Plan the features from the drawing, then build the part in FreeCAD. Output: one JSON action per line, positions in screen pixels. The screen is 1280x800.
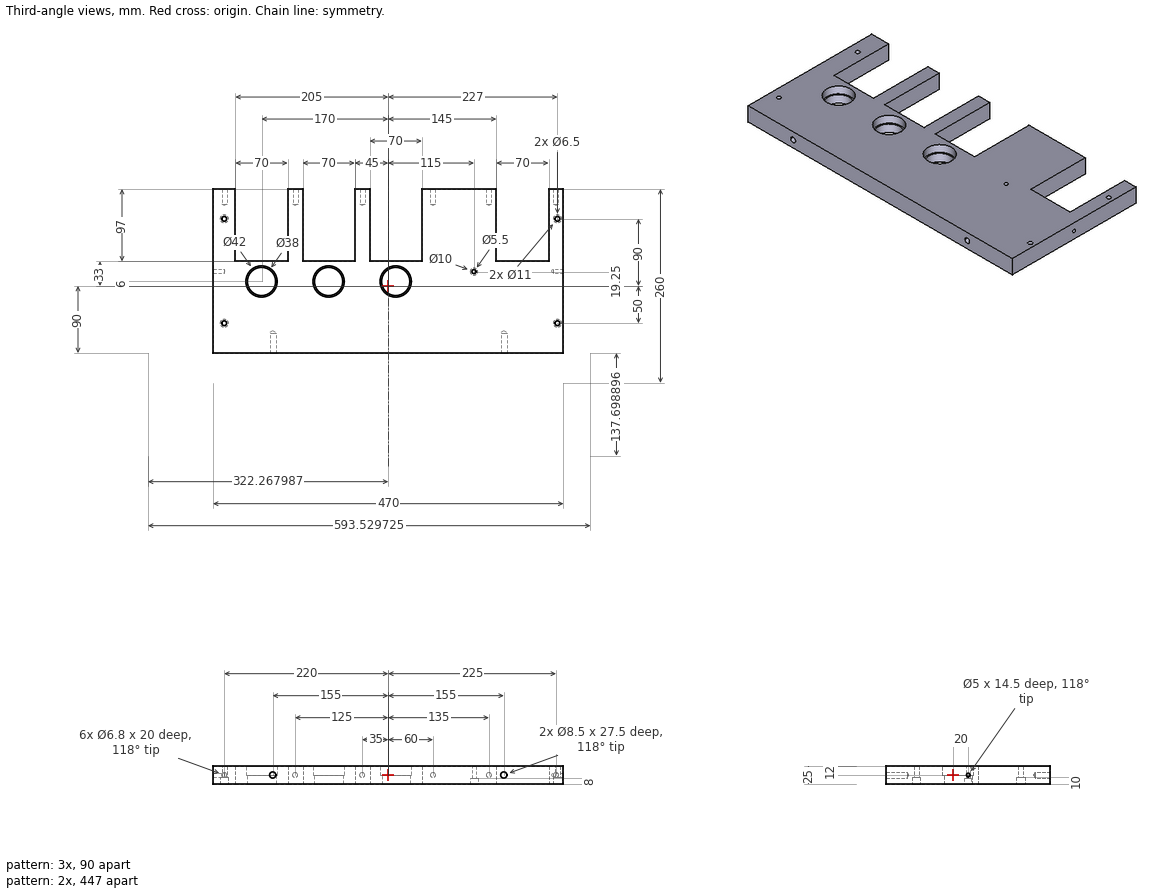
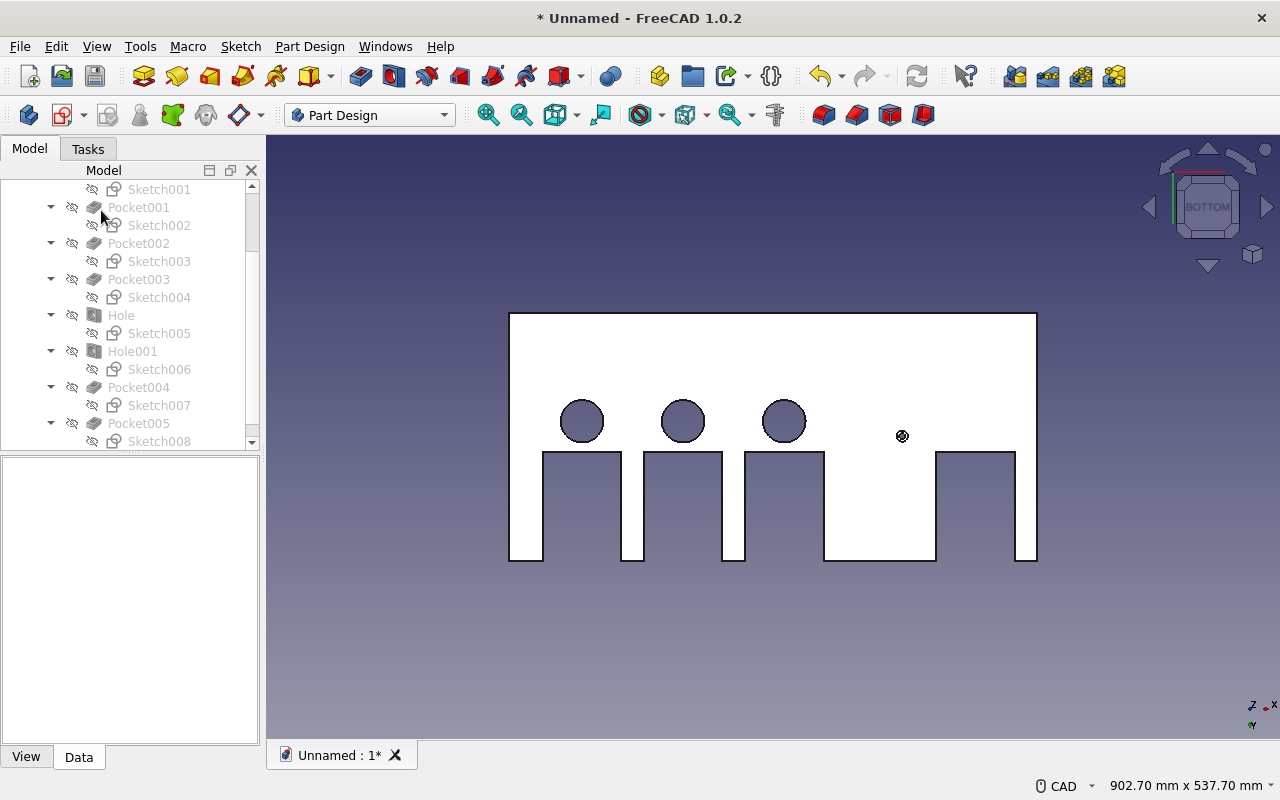
{"action": "left_click", "coordinate": [924, 365]}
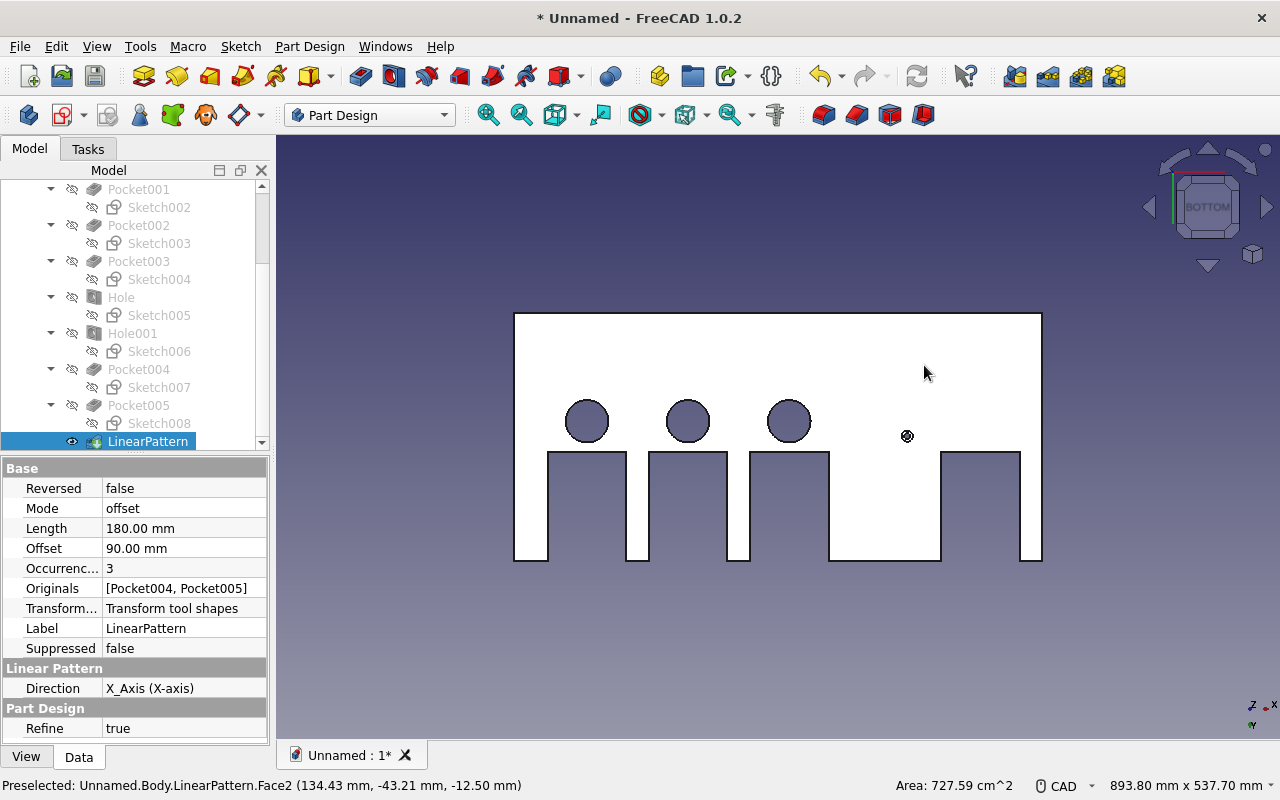
{"action": "left_click", "coordinate": [62, 116]}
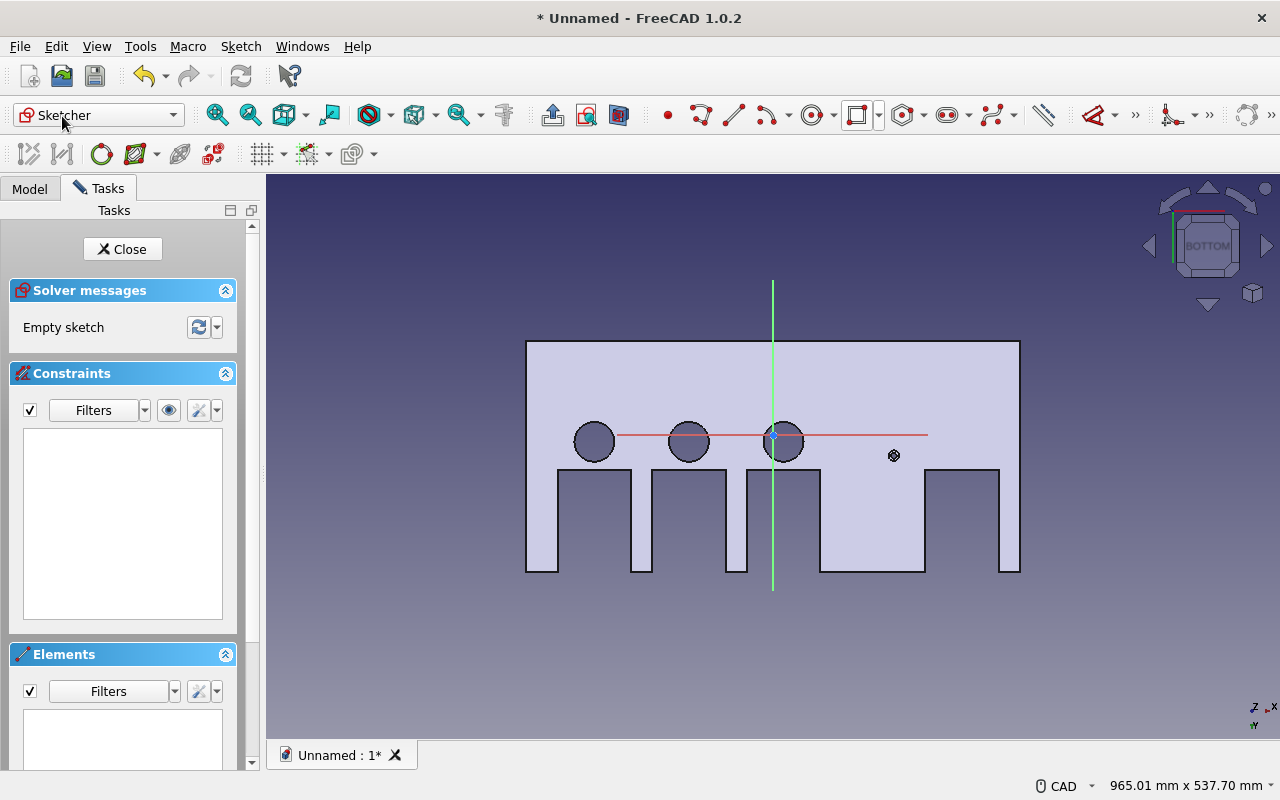
{"action": "scroll", "coordinate": [1049, 457], "scroll_direction": "up", "scroll_amount": 4}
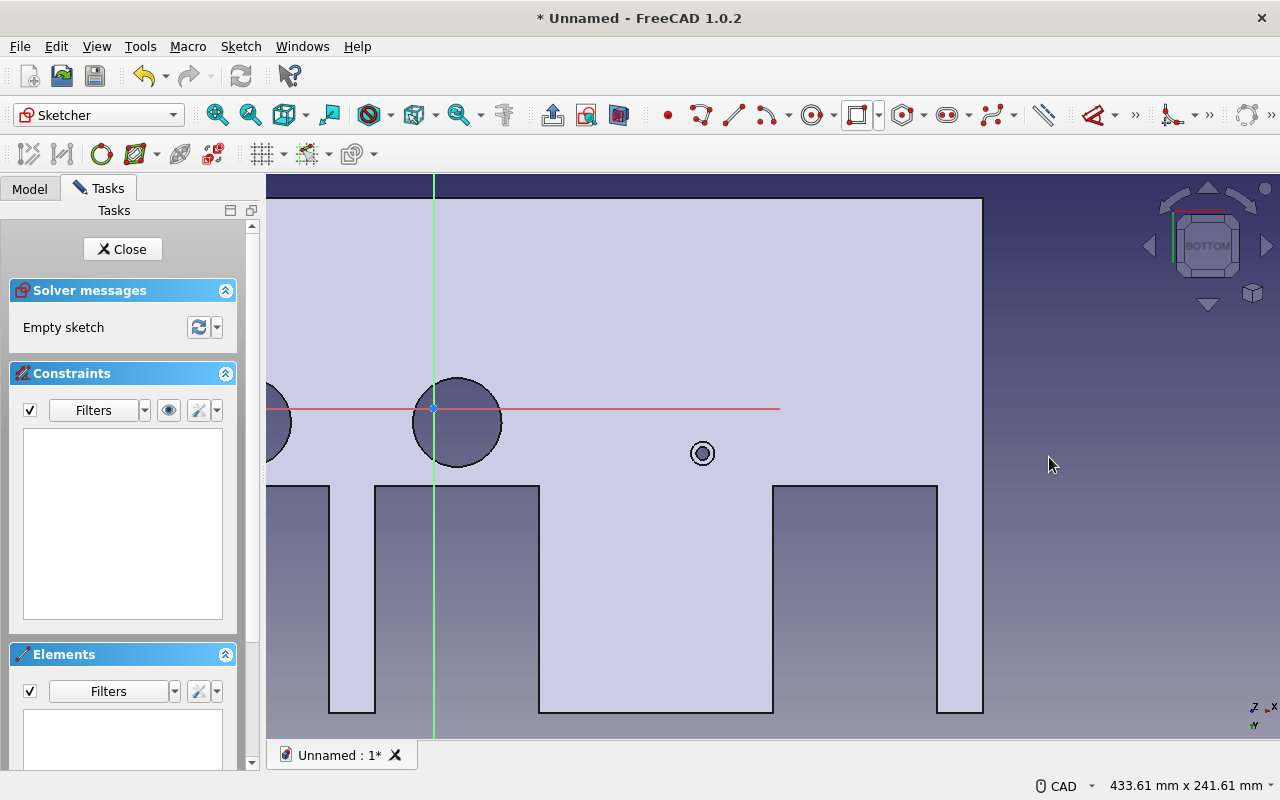
{"action": "left_click", "coordinate": [812, 116]}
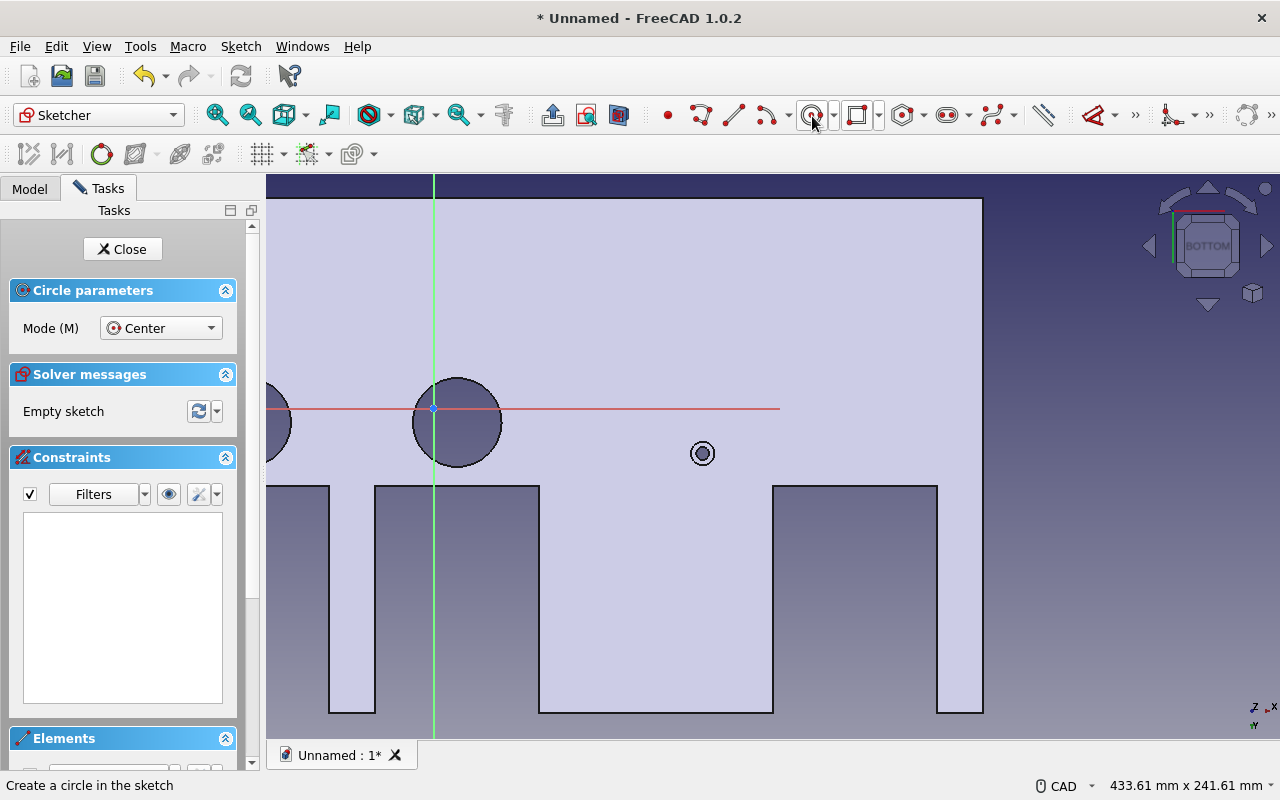
{"action": "scroll", "coordinate": [965, 619], "scroll_direction": "up", "scroll_amount": 6}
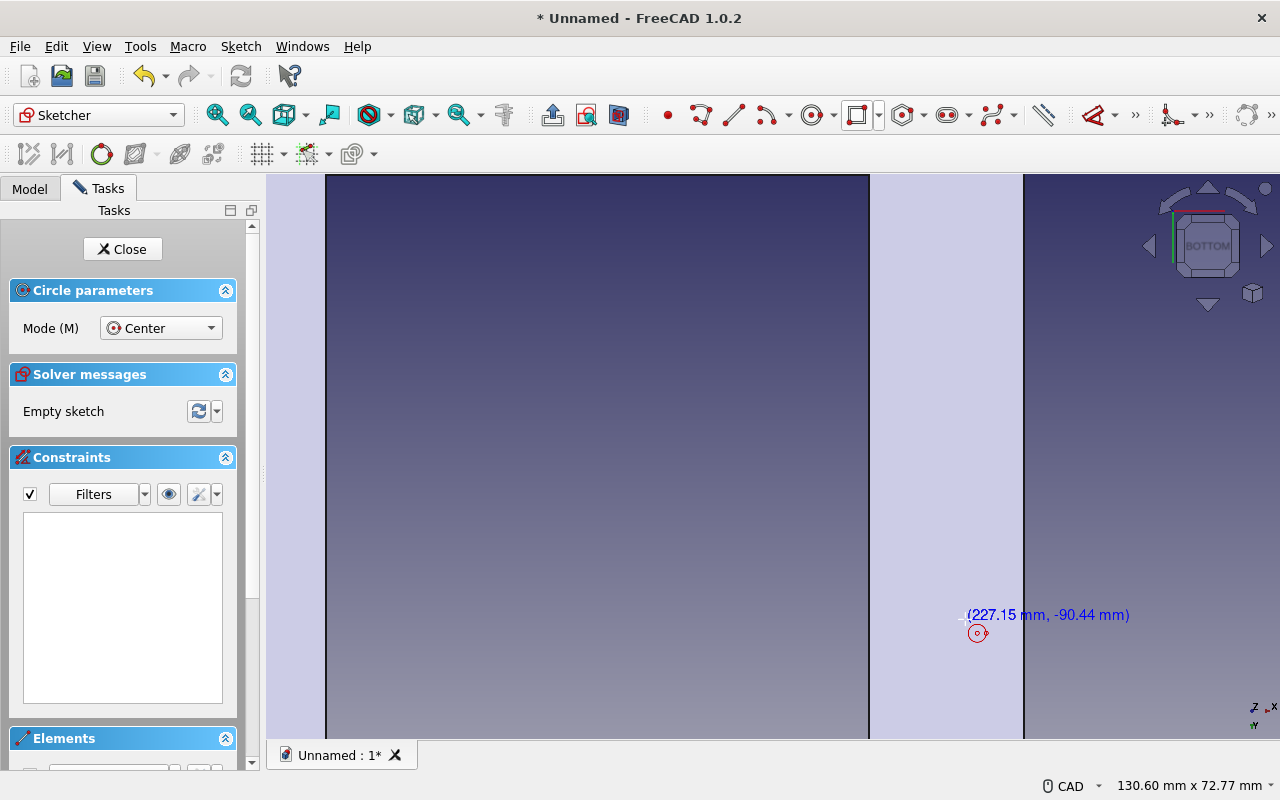
{"action": "left_click", "coordinate": [962, 617]}
{"action": "mouse_move", "coordinate": [980, 599]}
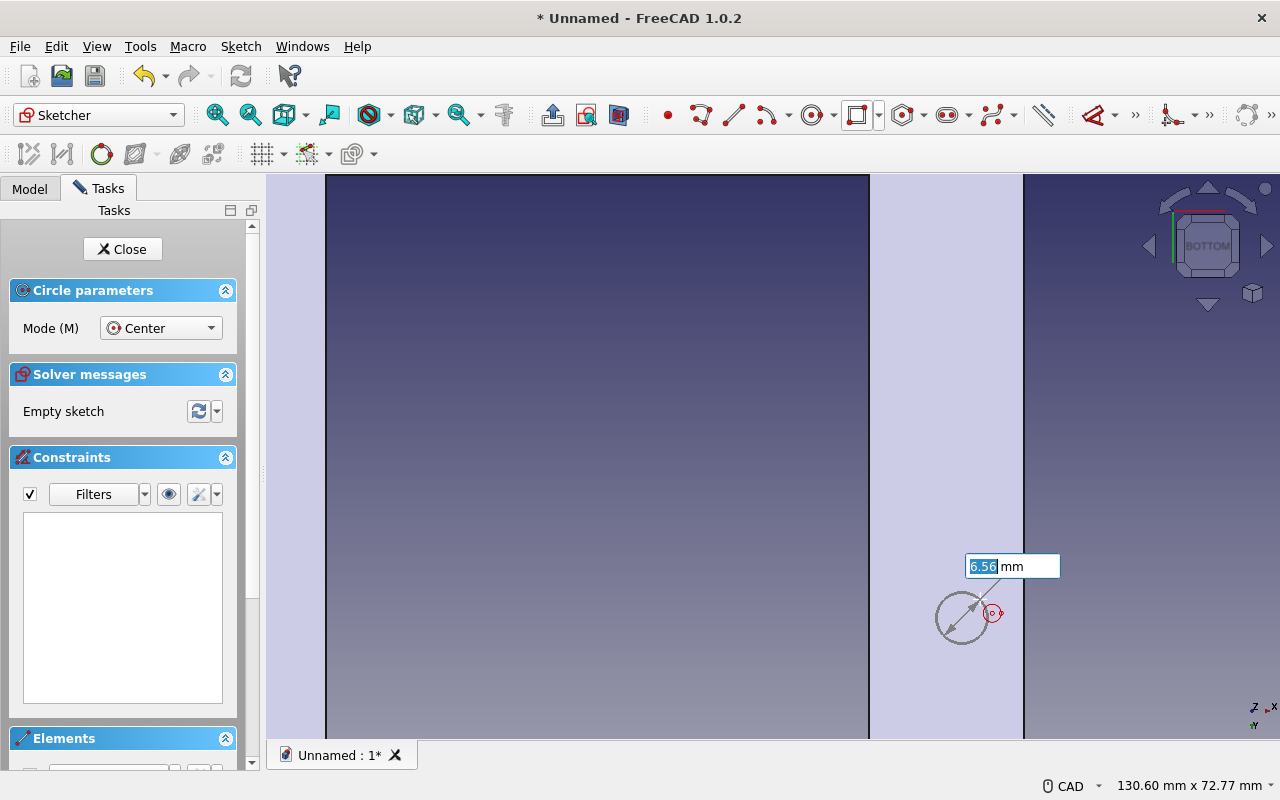
{"action": "type", "text": "6.5"}
{"action": "key", "text": "Return"}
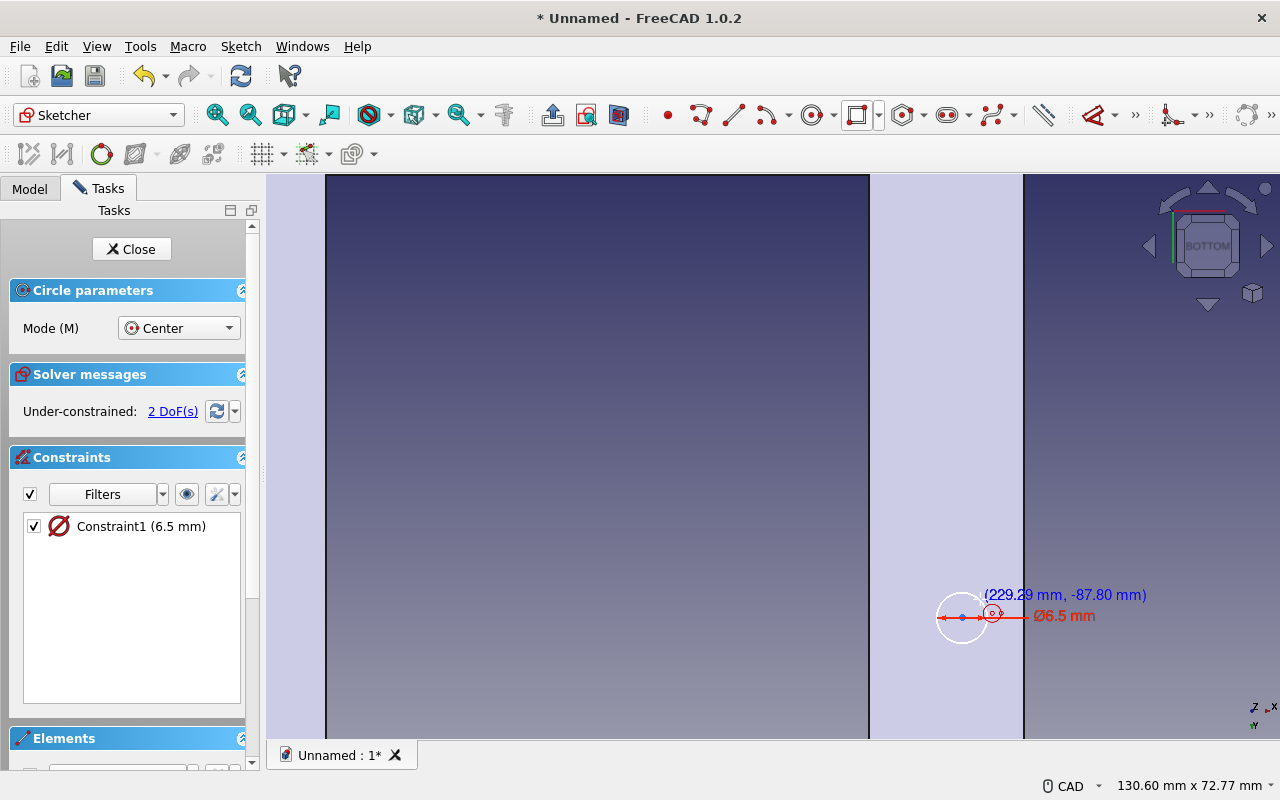
{"action": "scroll", "coordinate": [968, 622], "scroll_direction": "down", "scroll_amount": 6}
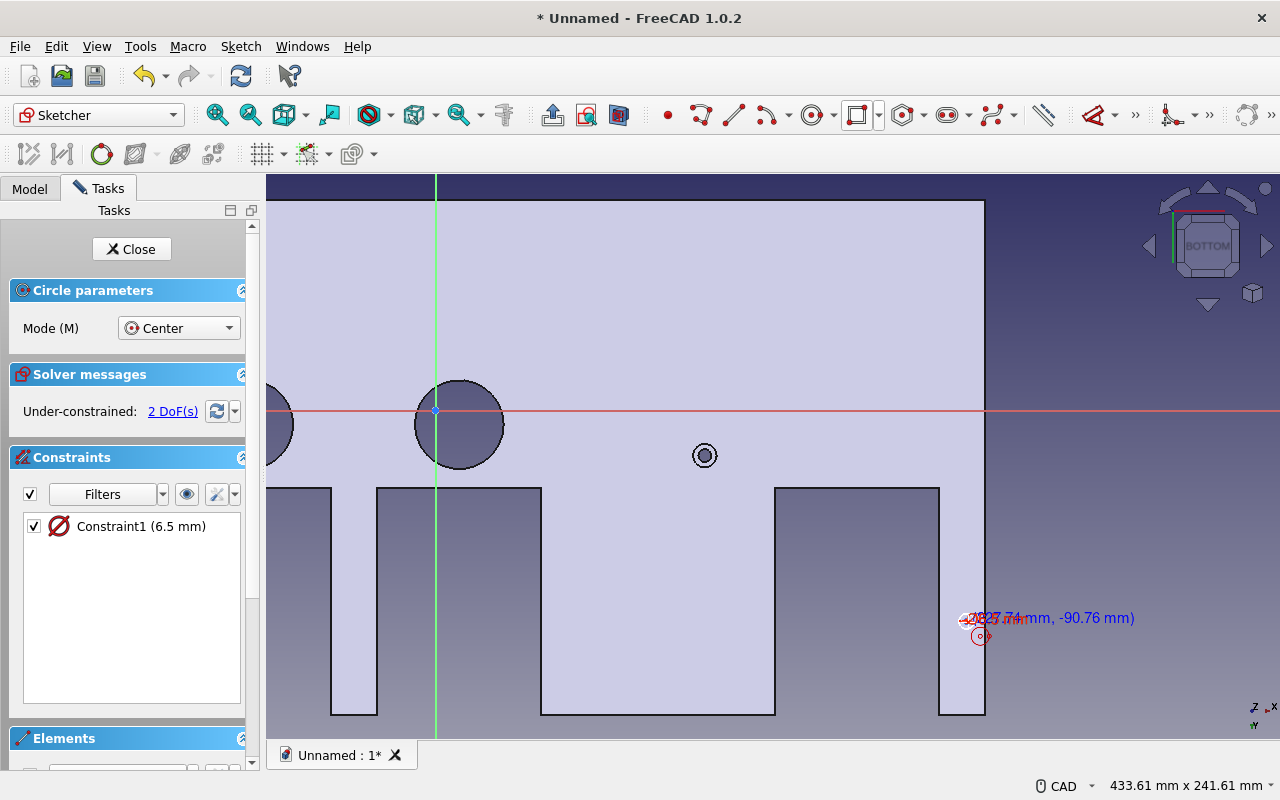
{"action": "scroll", "coordinate": [967, 294], "scroll_direction": "up", "scroll_amount": 6}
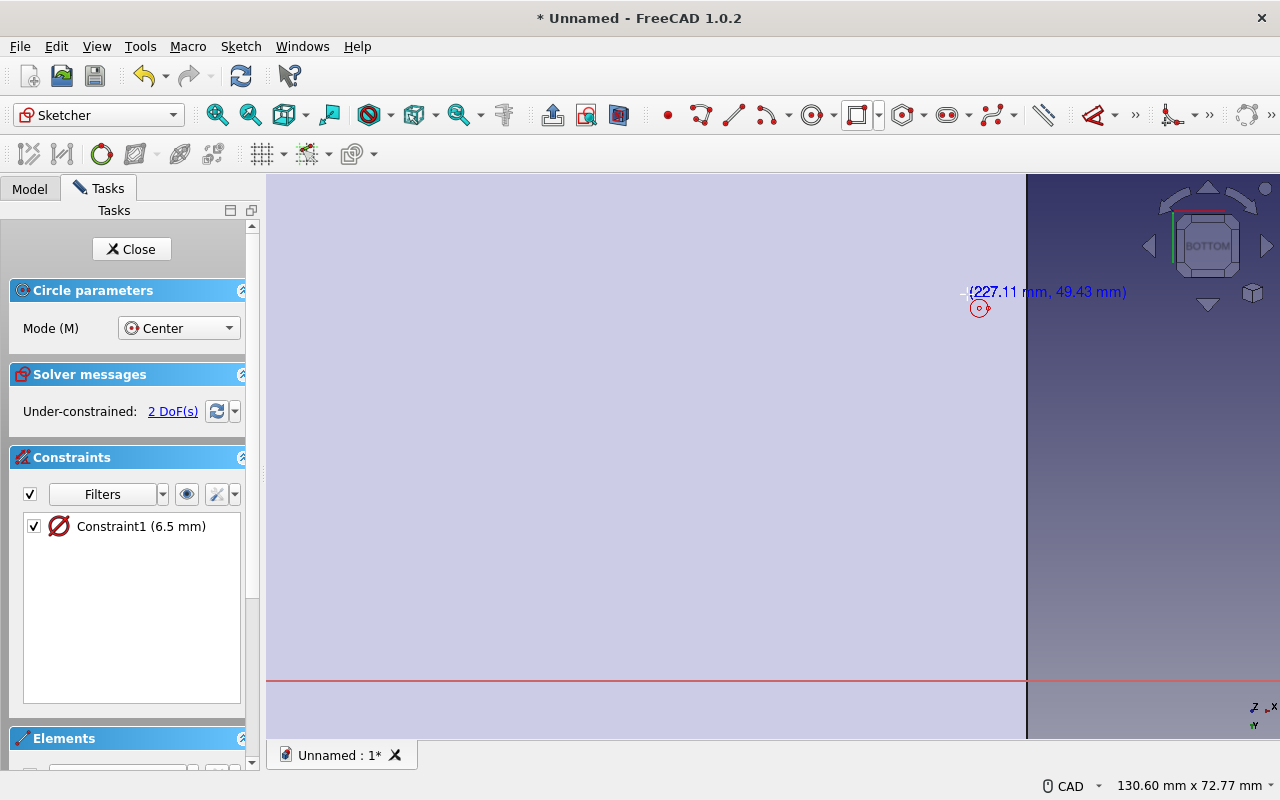
{"action": "left_click", "coordinate": [965, 292]}
{"action": "mouse_move", "coordinate": [982, 275]}